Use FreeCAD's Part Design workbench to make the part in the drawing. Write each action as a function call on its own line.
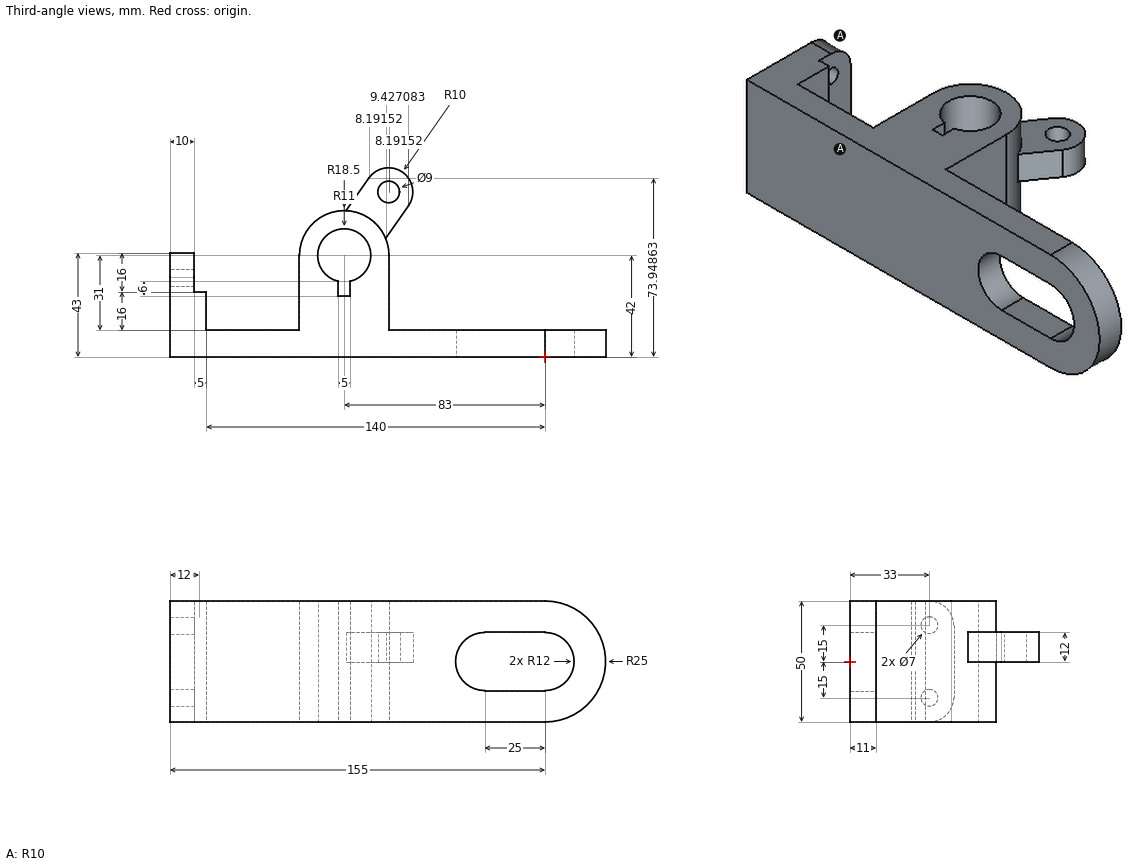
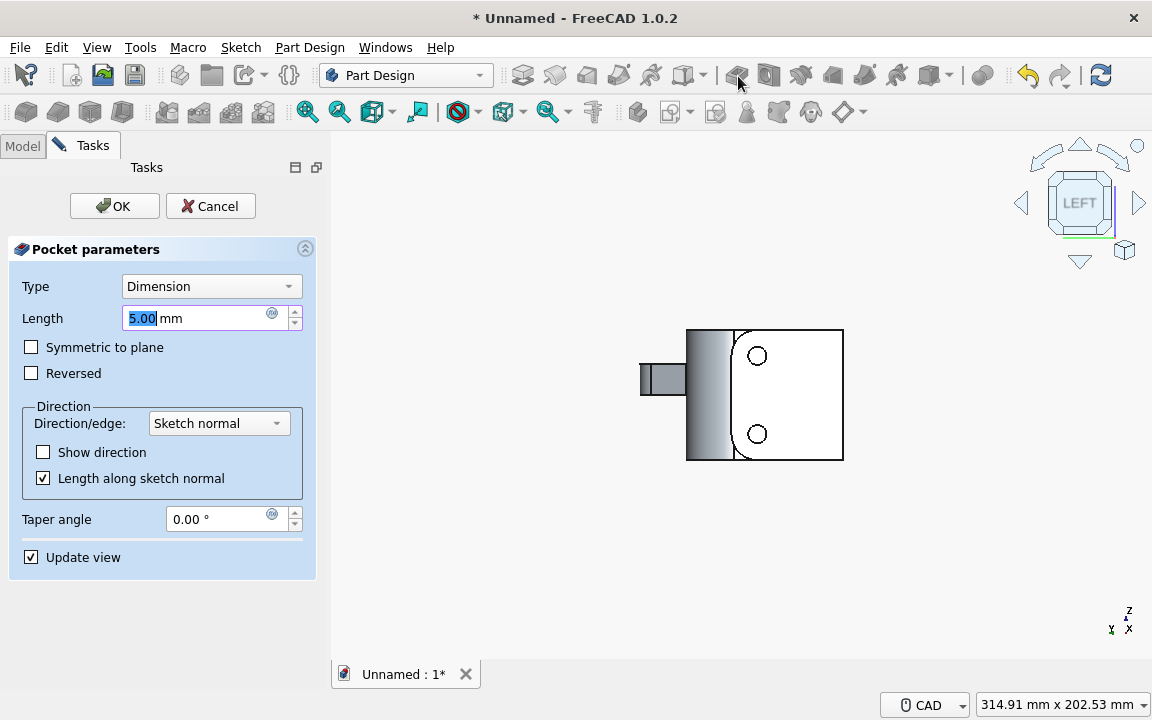
text(12)
key(Tab)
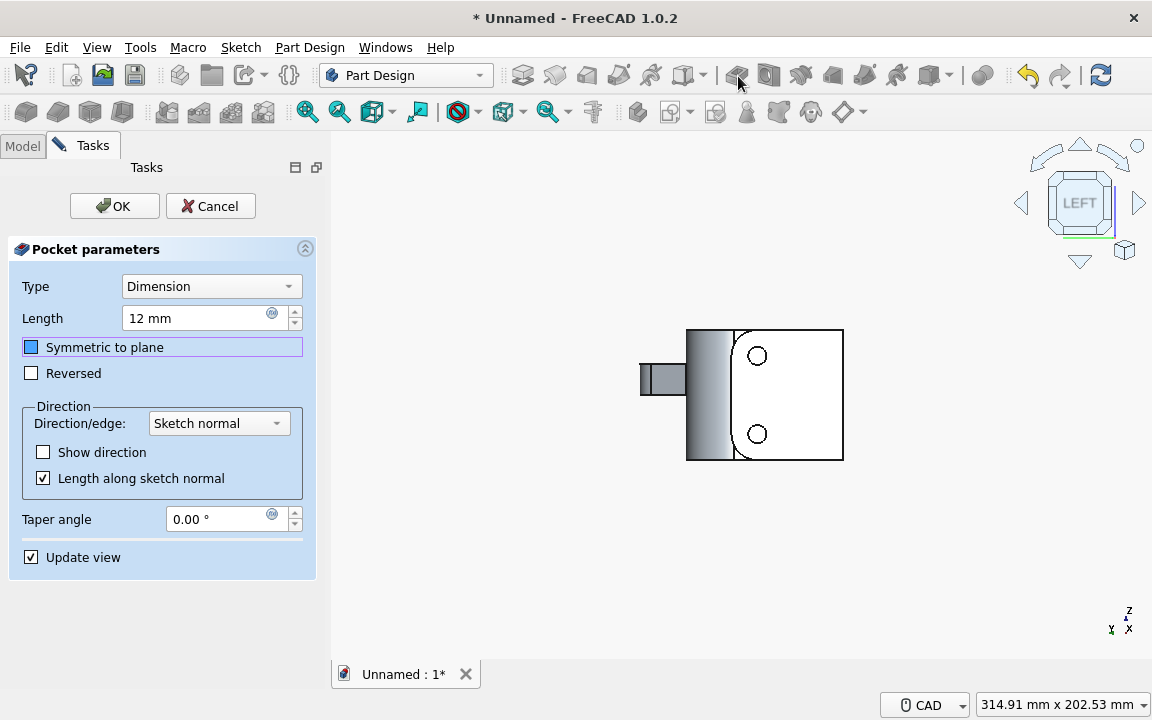
click(115, 206)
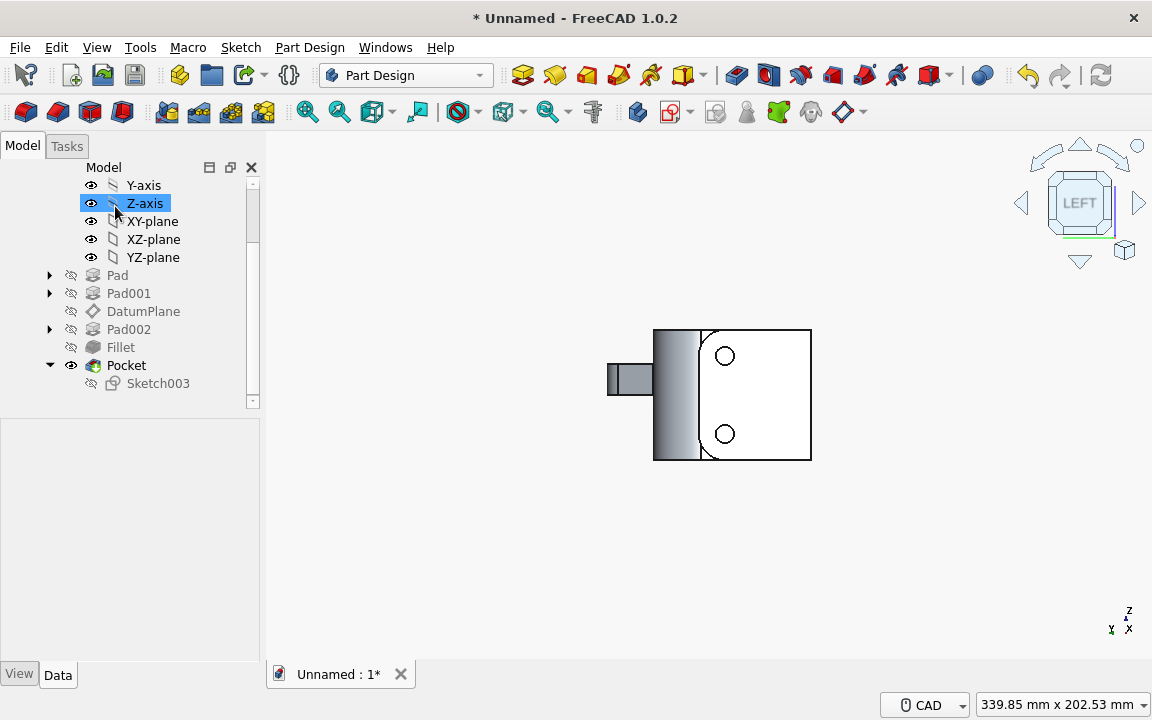
key(0)